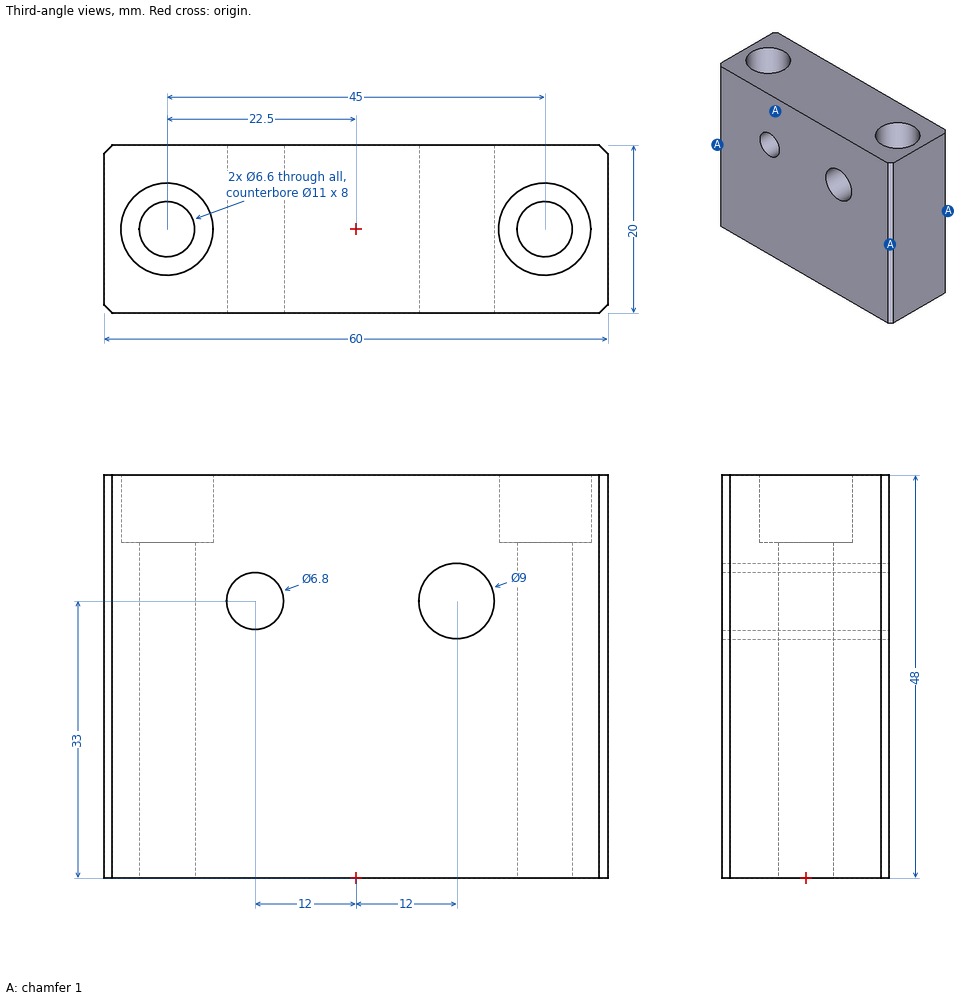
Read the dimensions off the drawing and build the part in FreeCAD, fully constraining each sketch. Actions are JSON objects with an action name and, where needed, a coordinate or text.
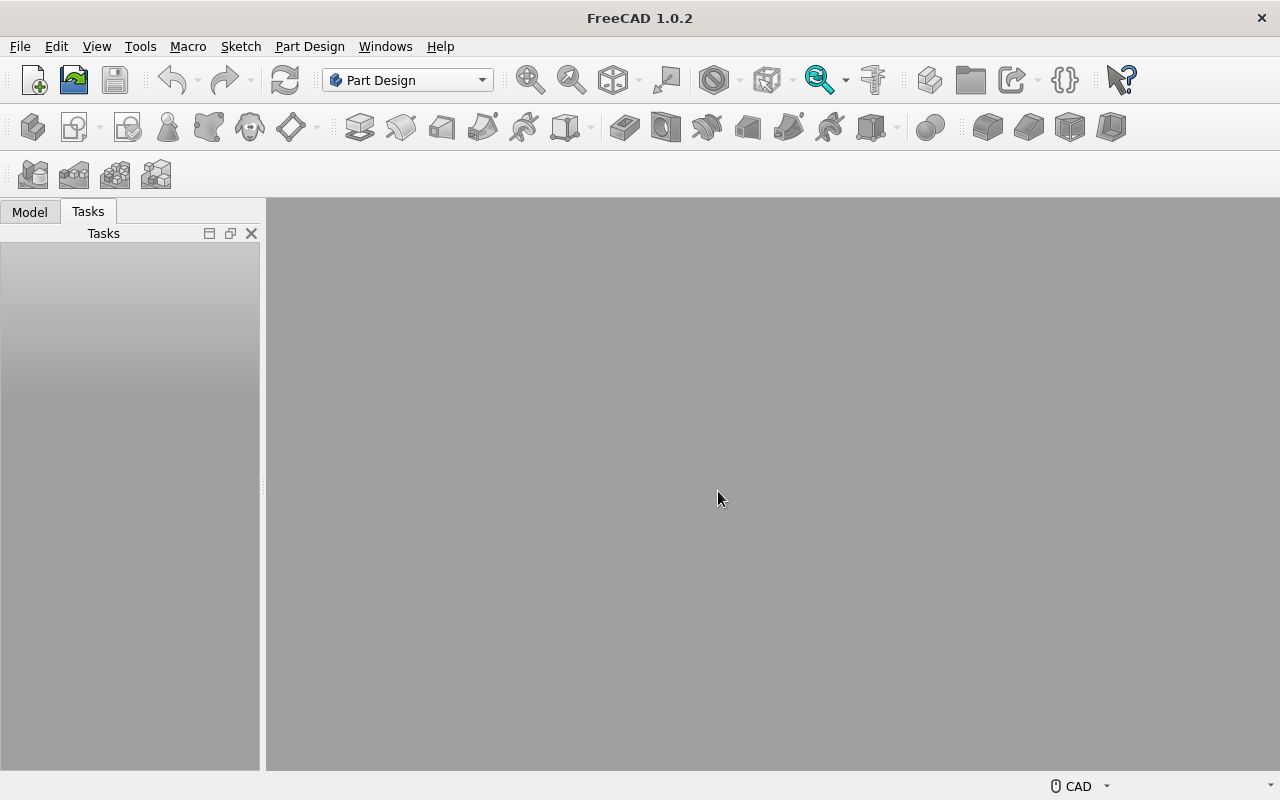
{"action": "key", "text": "ctrl+n"}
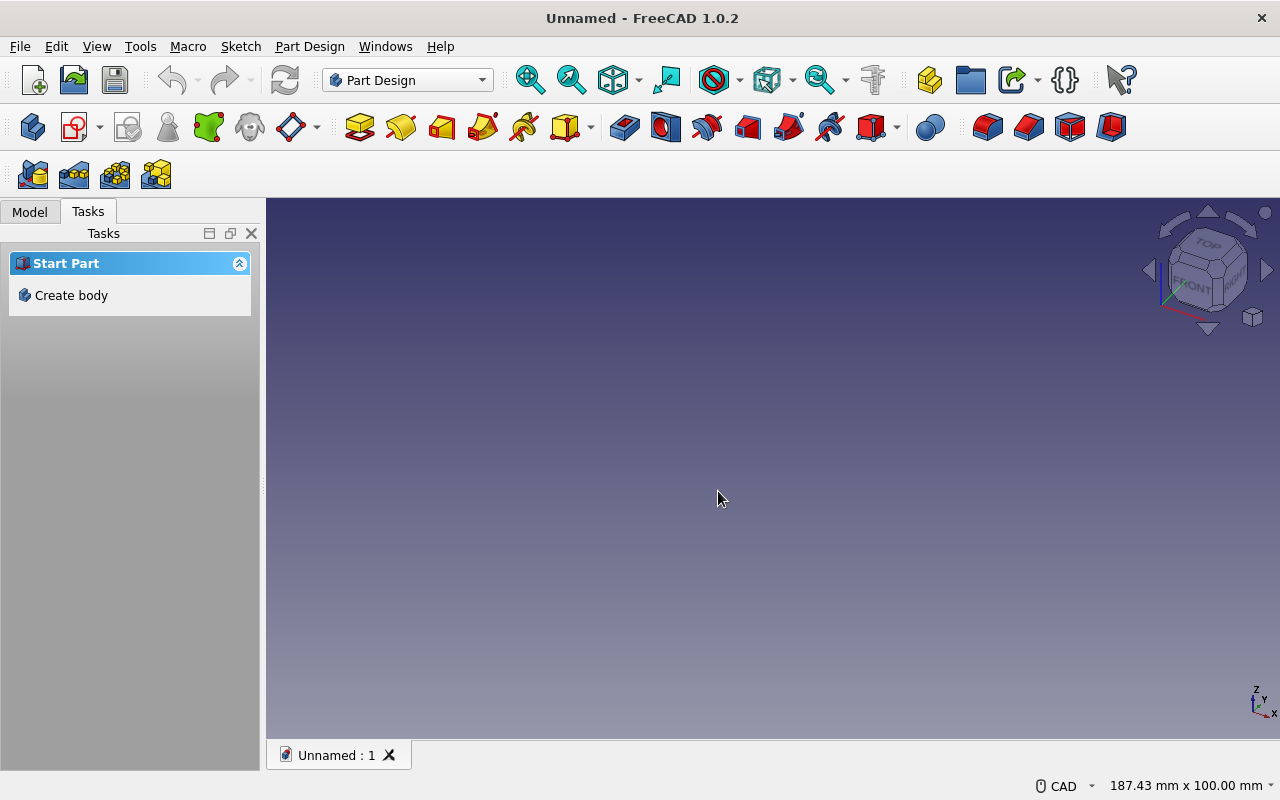
{"action": "left_click", "coordinate": [74, 128]}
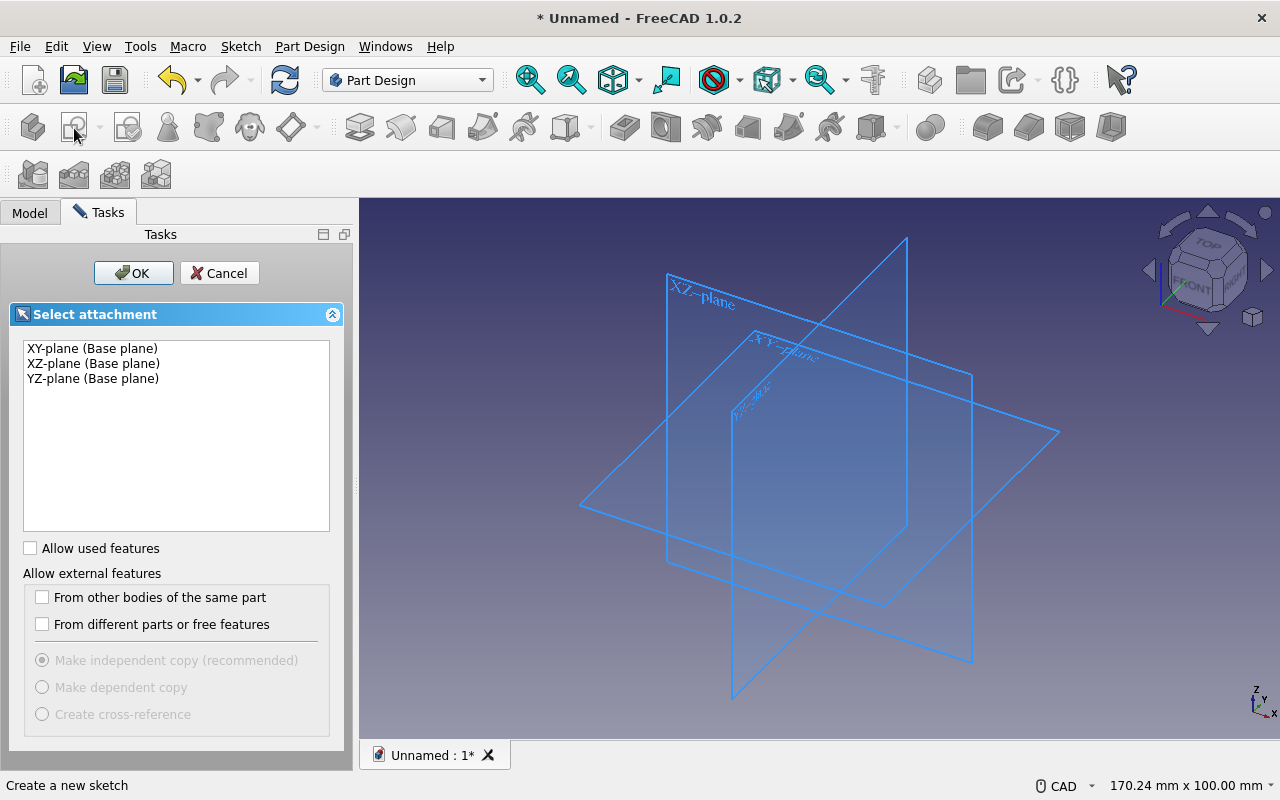
{"action": "left_click", "coordinate": [84, 348]}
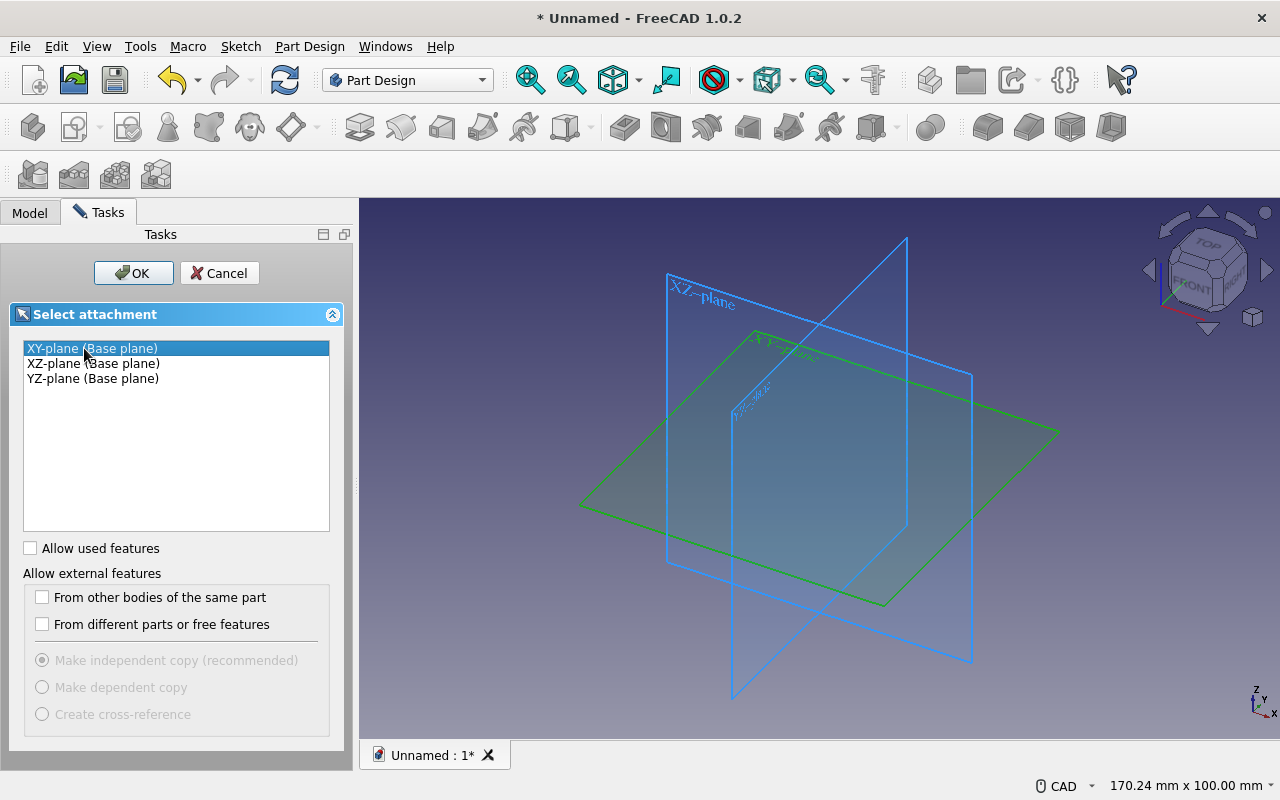
{"action": "left_click", "coordinate": [134, 273]}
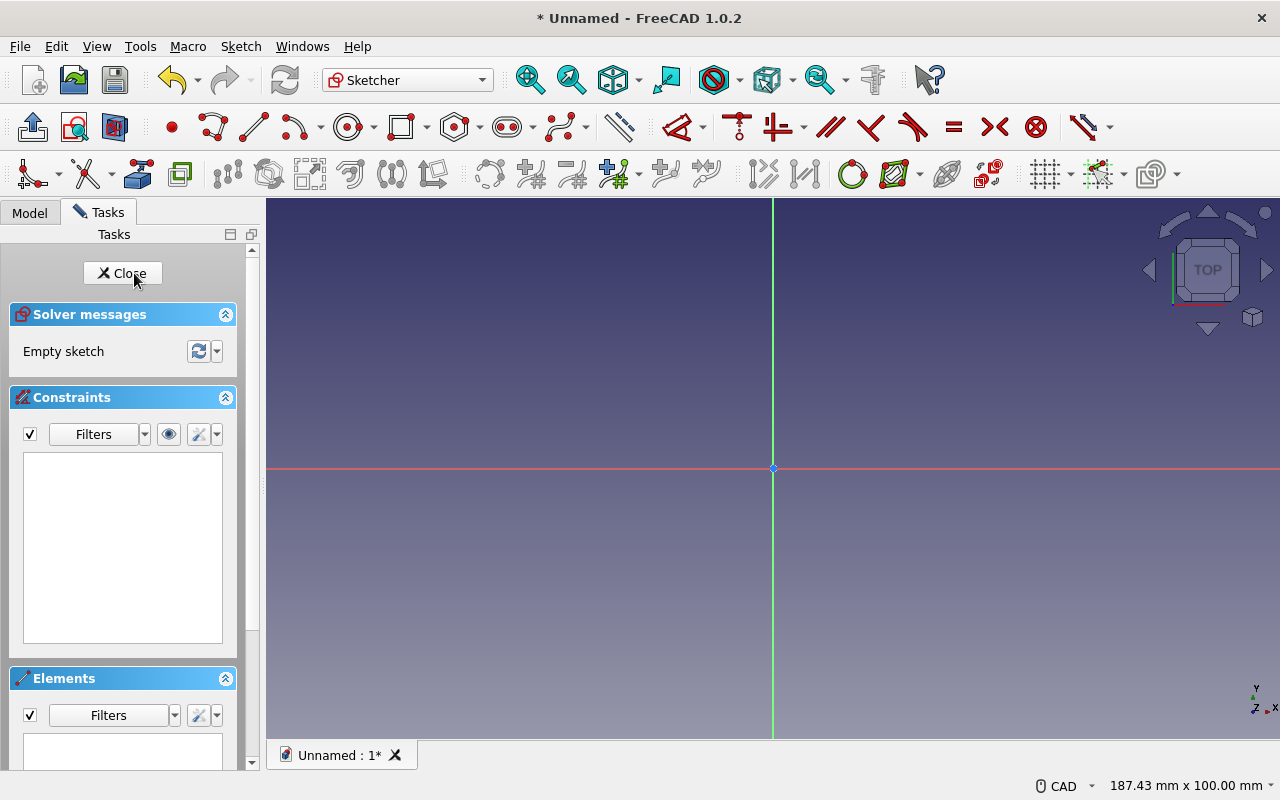
{"action": "scroll", "coordinate": [856, 468], "scroll_direction": "up", "scroll_amount": 3}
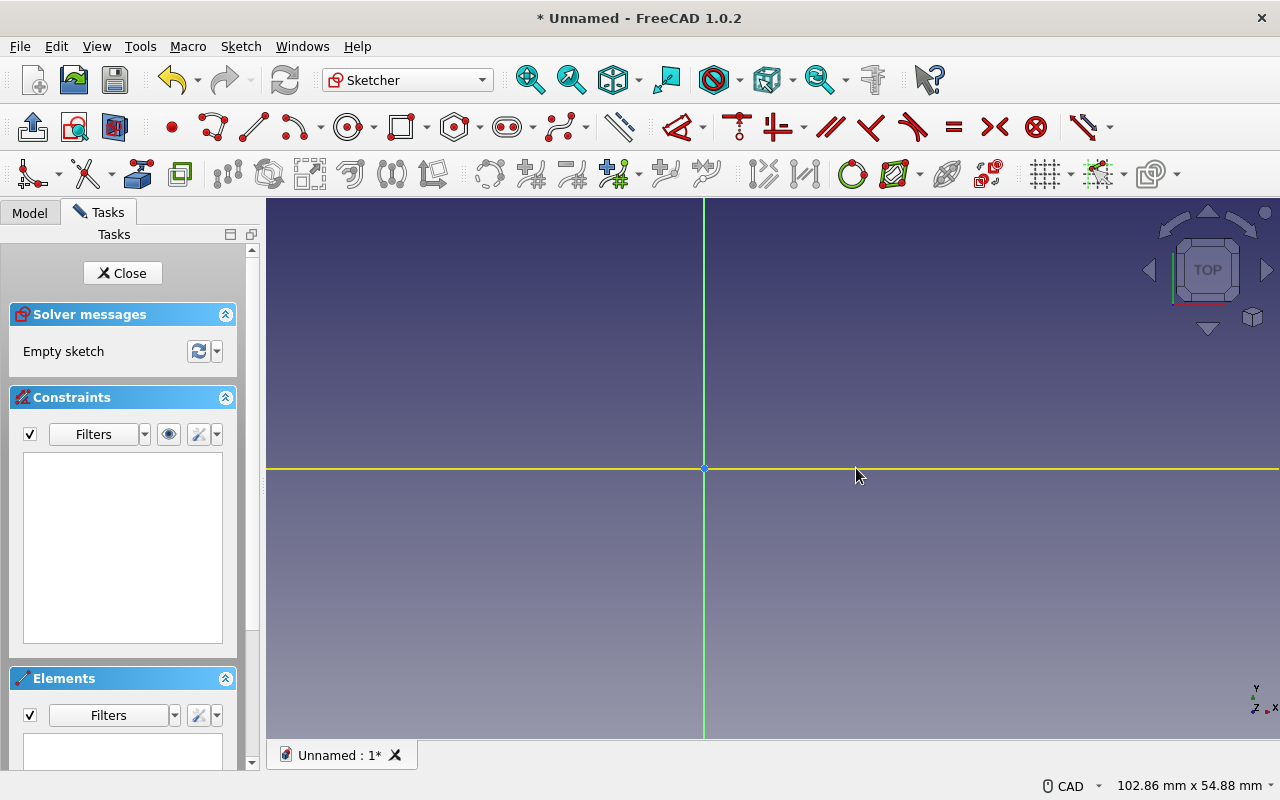
{"action": "left_click", "coordinate": [426, 128]}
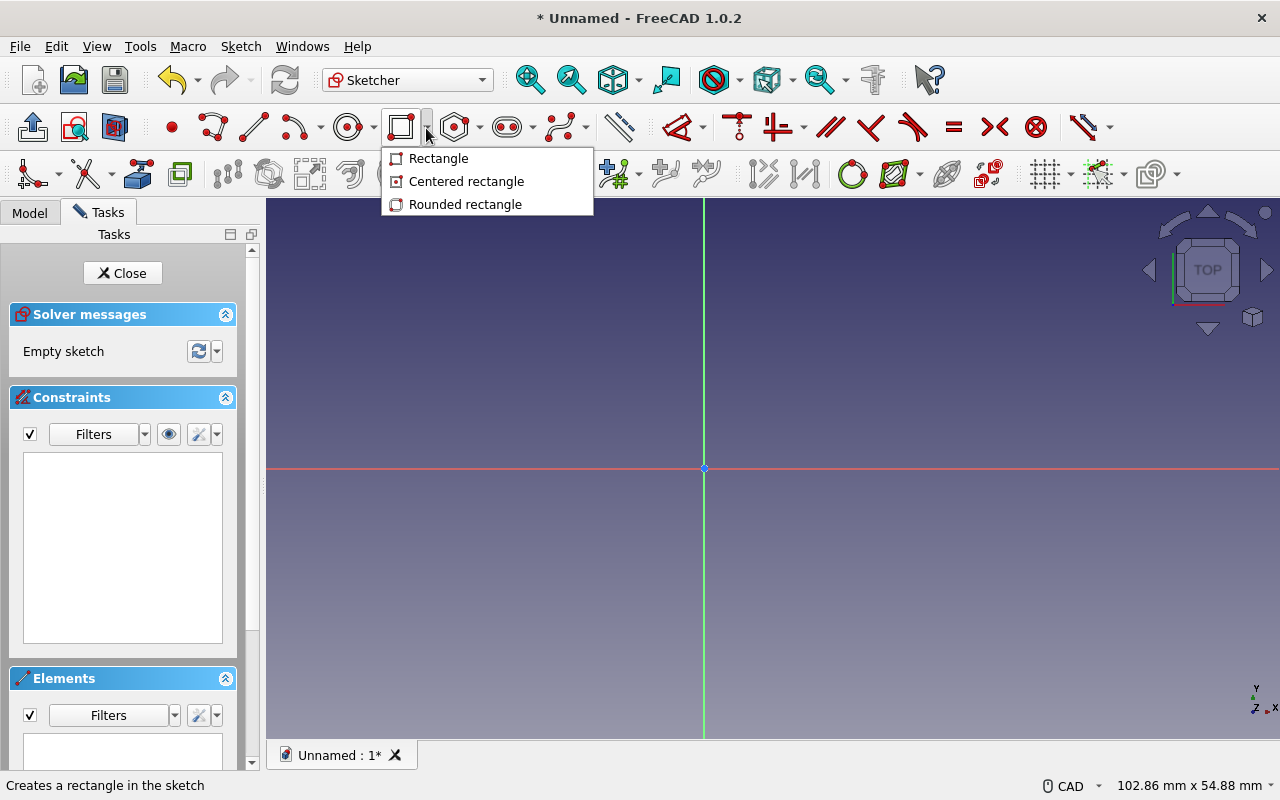
{"action": "left_click", "coordinate": [488, 182]}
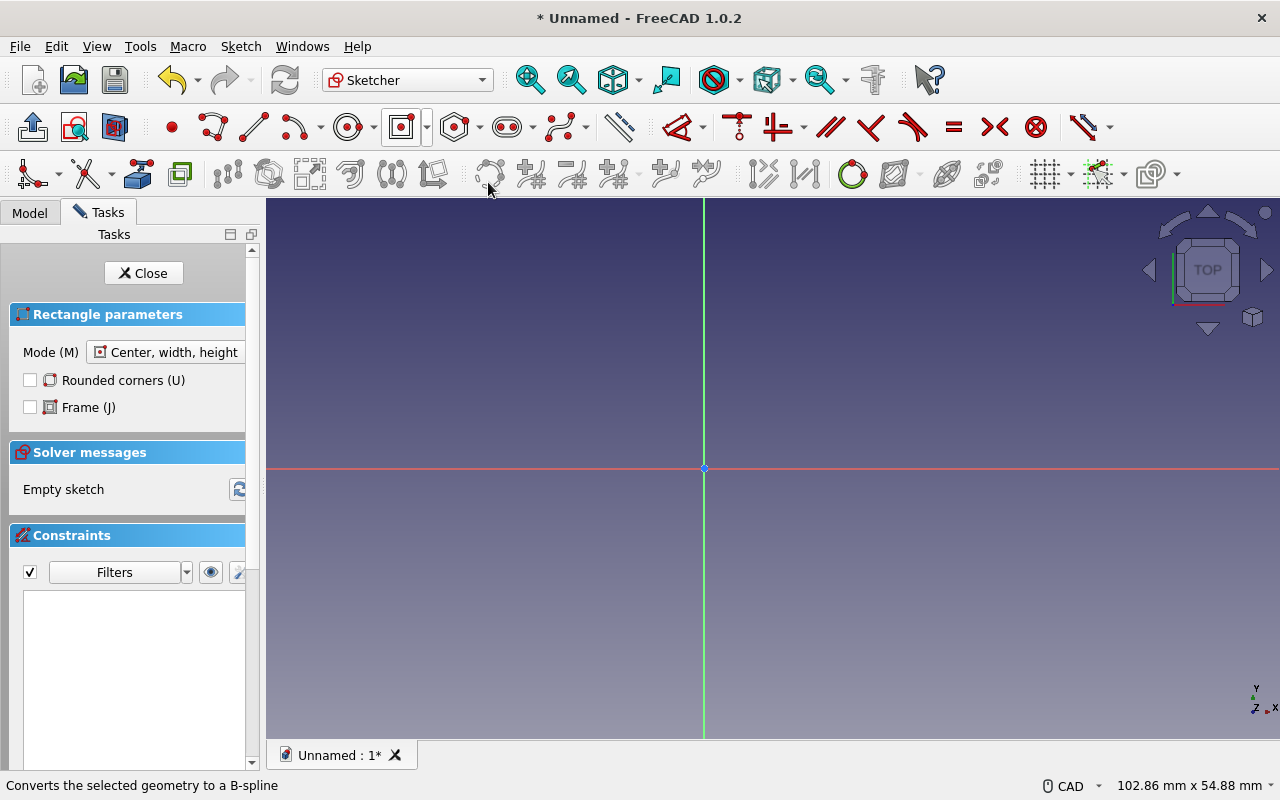
{"action": "left_click", "coordinate": [704, 468]}
{"action": "mouse_move", "coordinate": [1000, 370]}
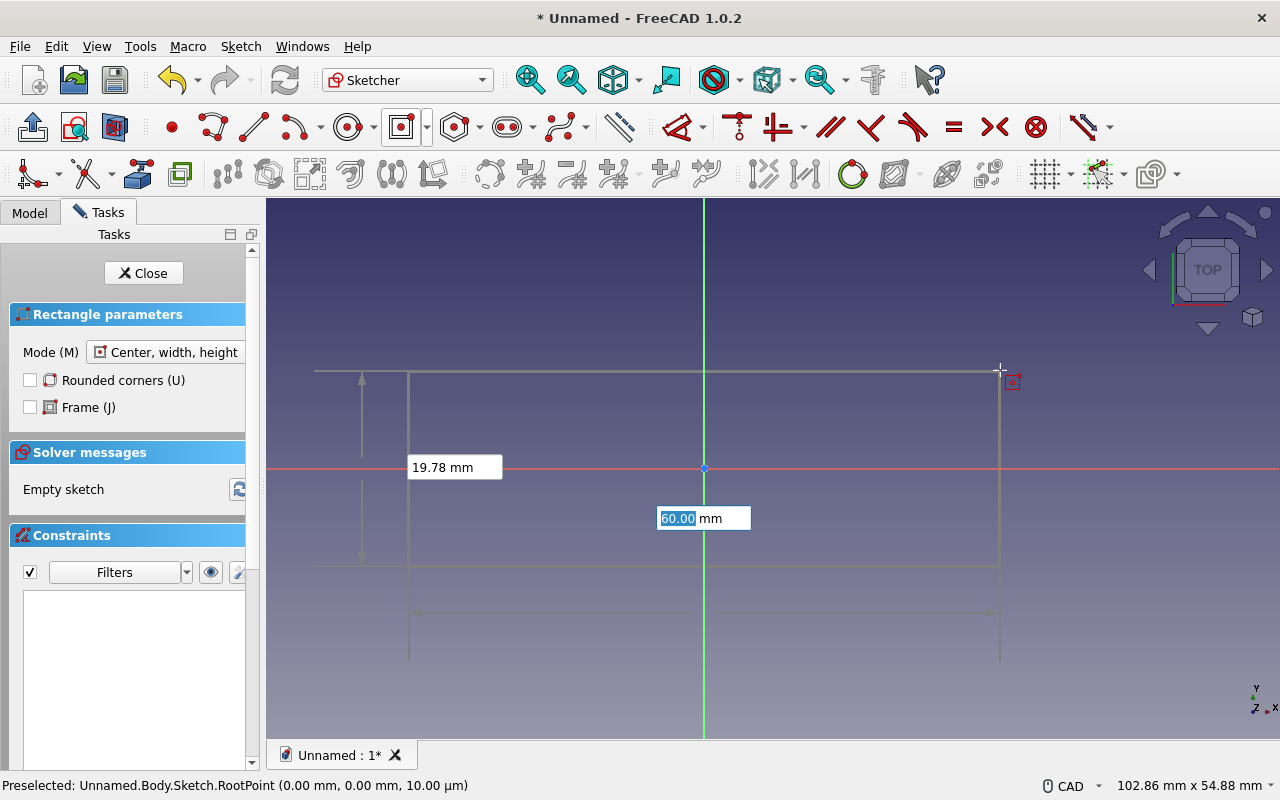
{"action": "type", "text": "60"}
{"action": "key", "text": "Tab"}
{"action": "type", "text": "20"}
{"action": "key", "text": "Return"}
{"action": "key", "text": "Escape"}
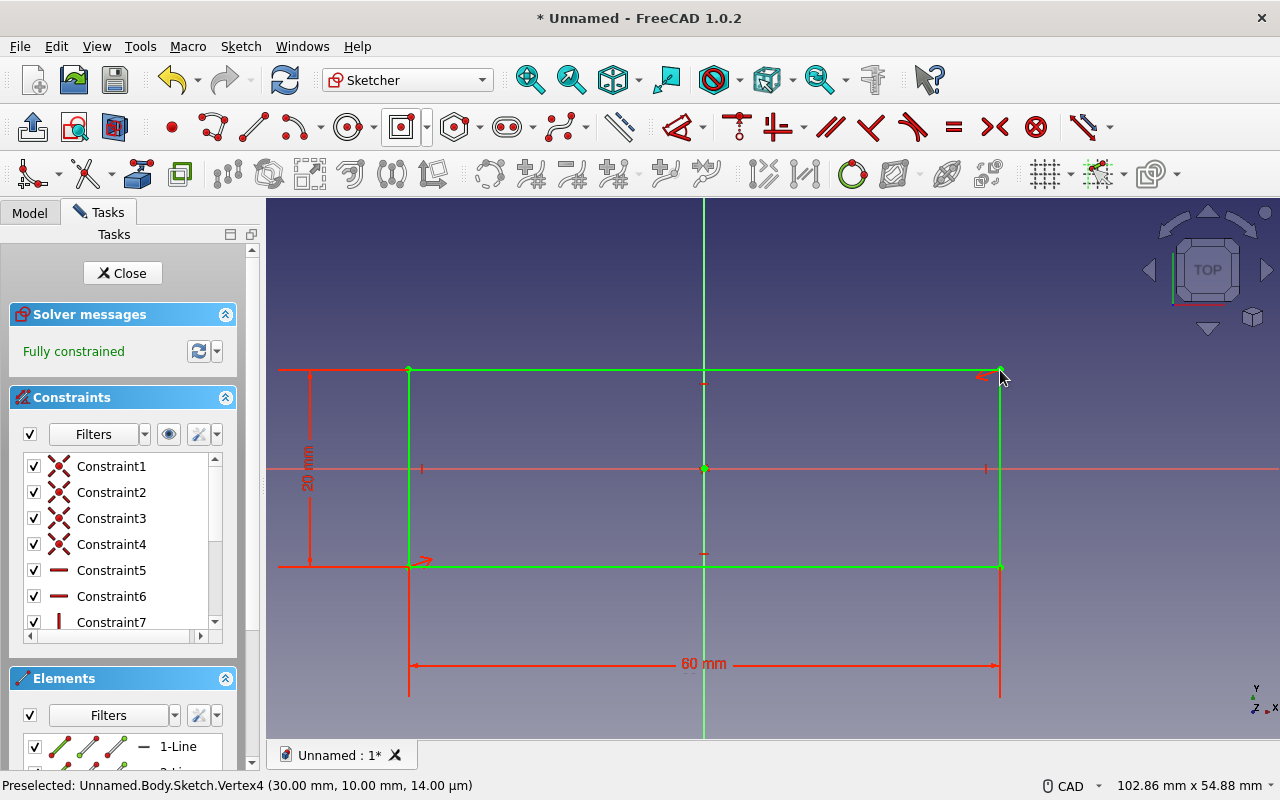
{"action": "left_click", "coordinate": [123, 273]}